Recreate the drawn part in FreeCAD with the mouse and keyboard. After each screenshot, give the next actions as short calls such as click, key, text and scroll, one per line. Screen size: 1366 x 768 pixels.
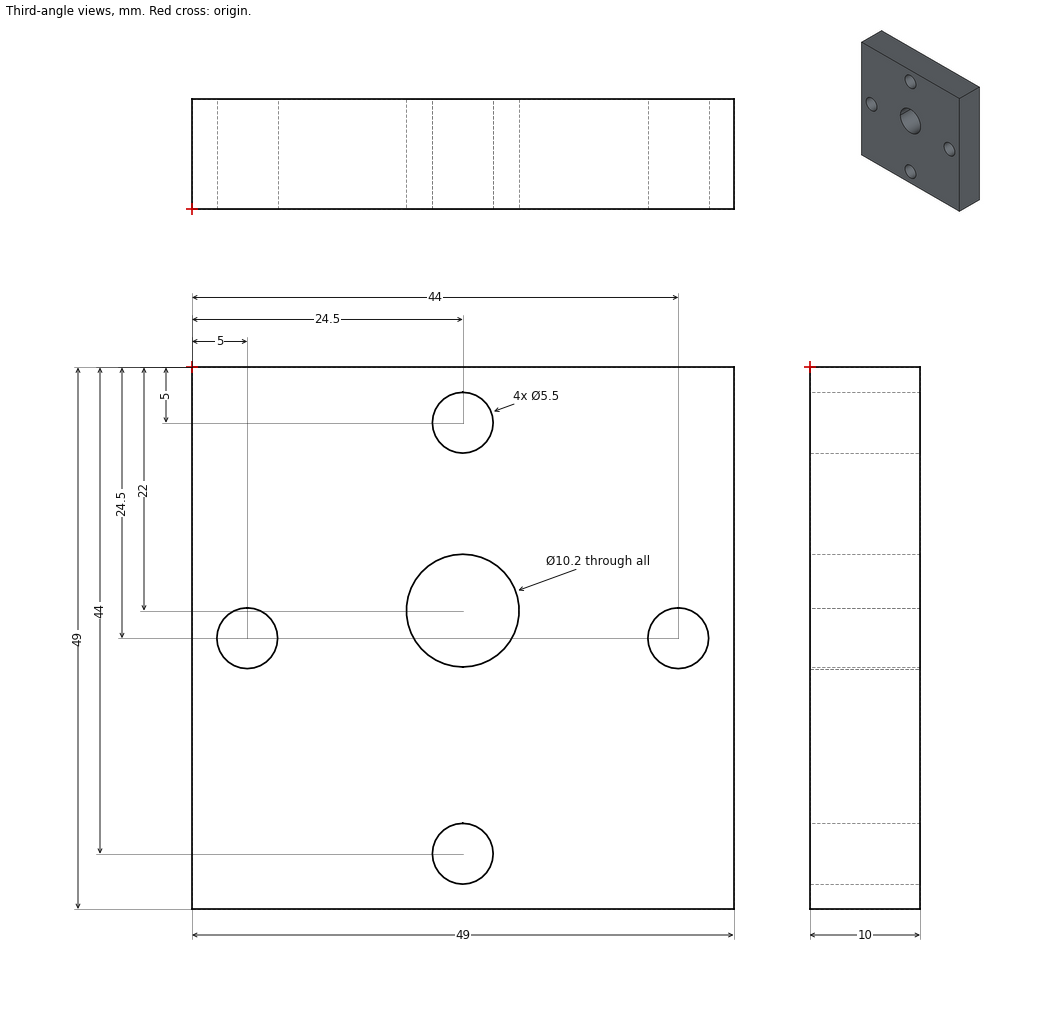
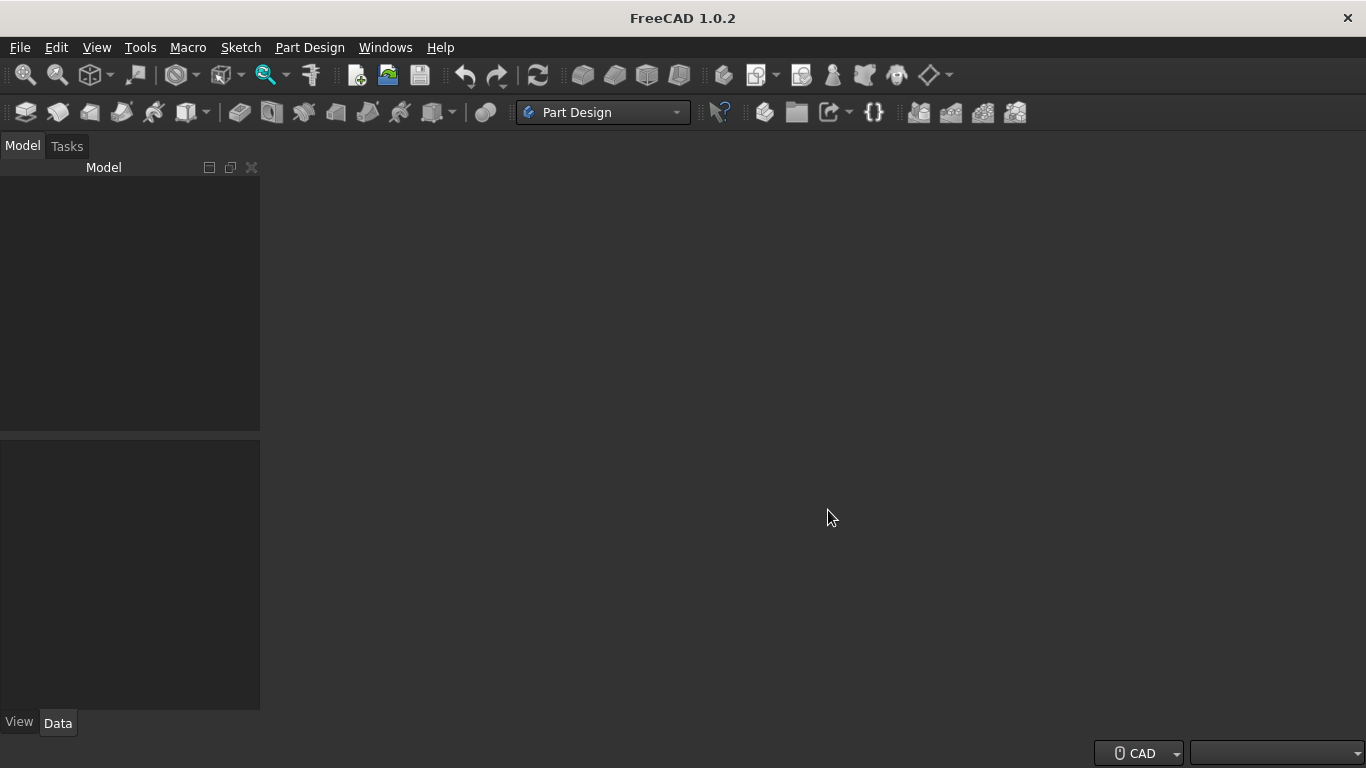
click(356, 76)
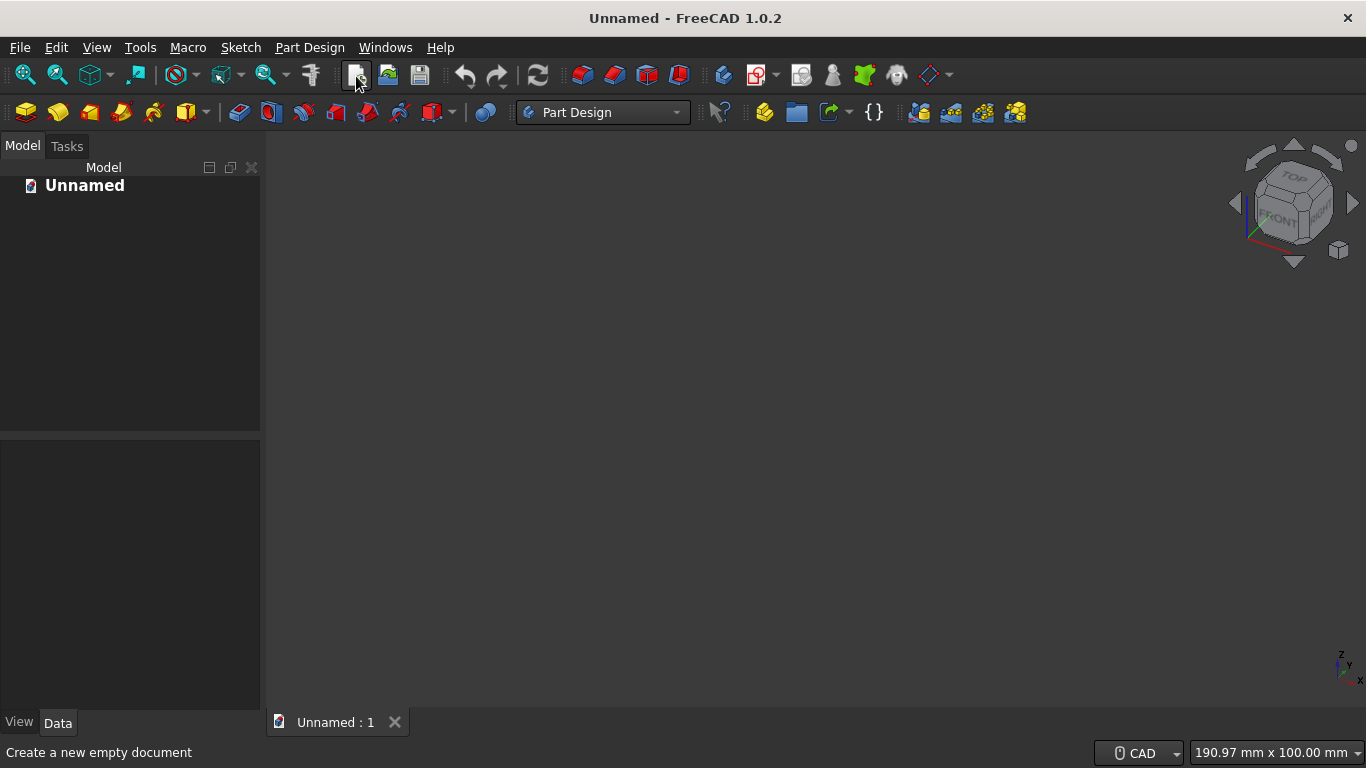
click(756, 76)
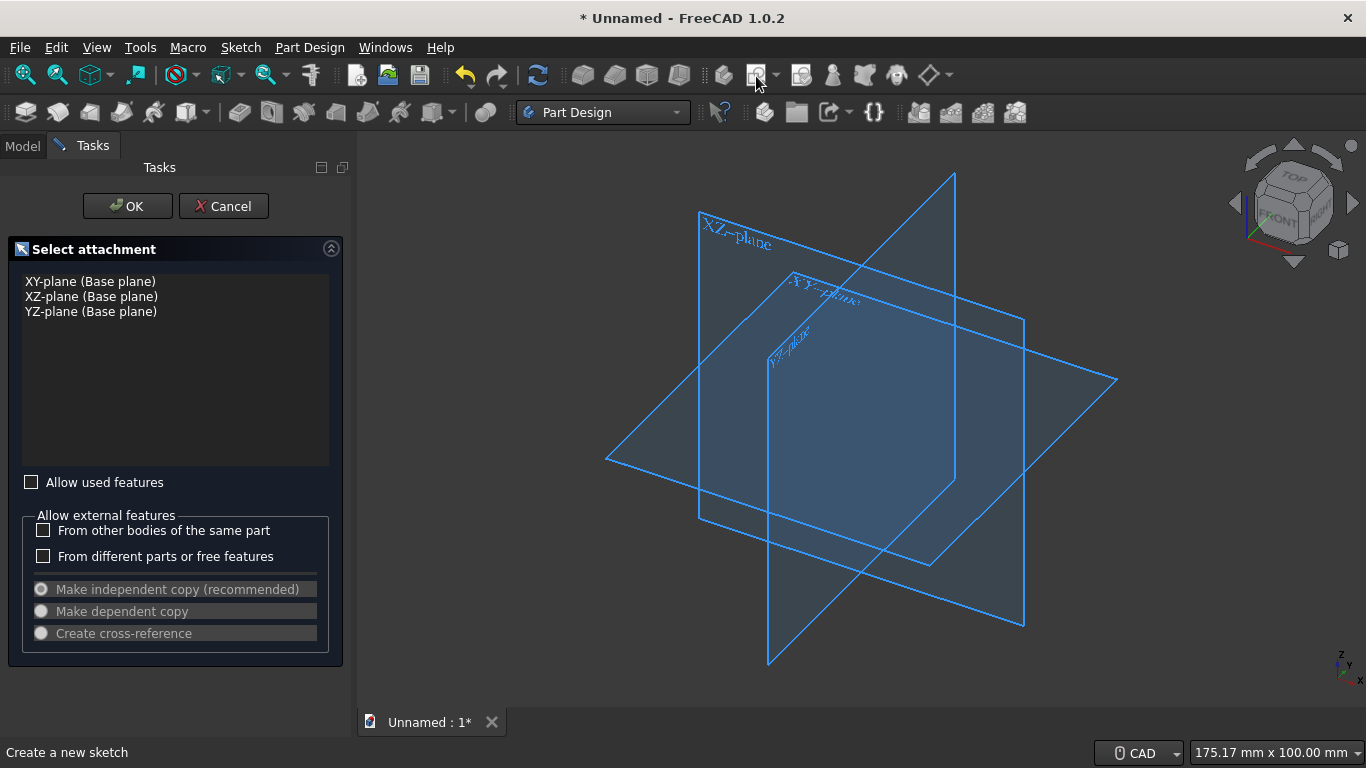
click(82, 296)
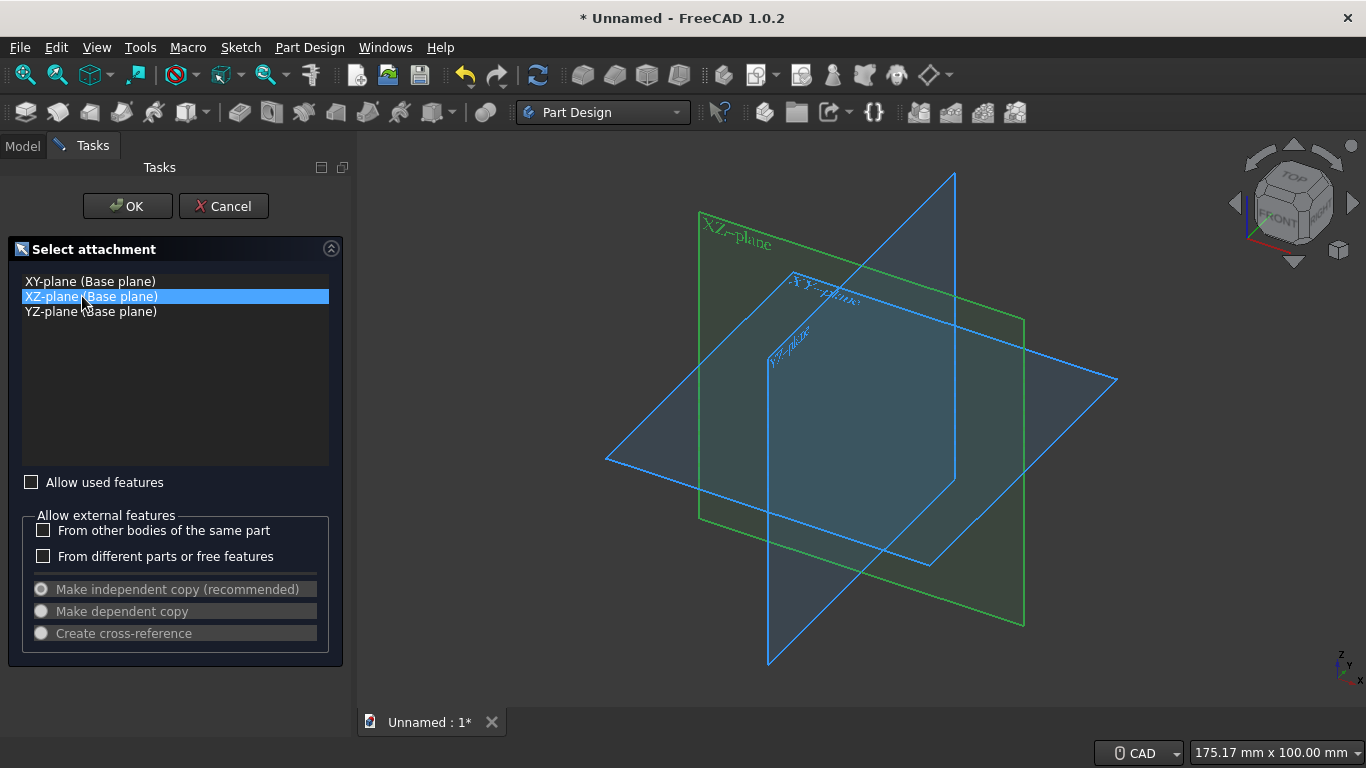
click(128, 206)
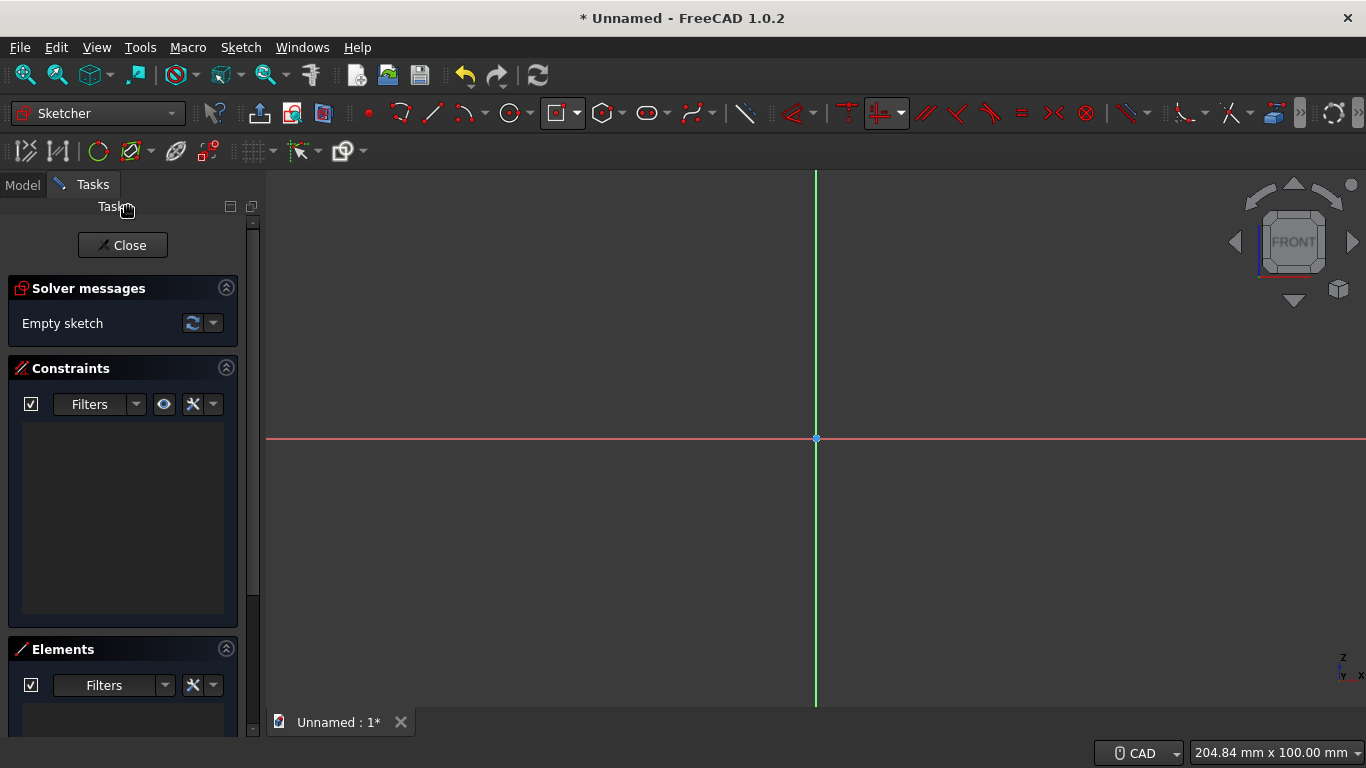
scroll(294, 198, down, 1)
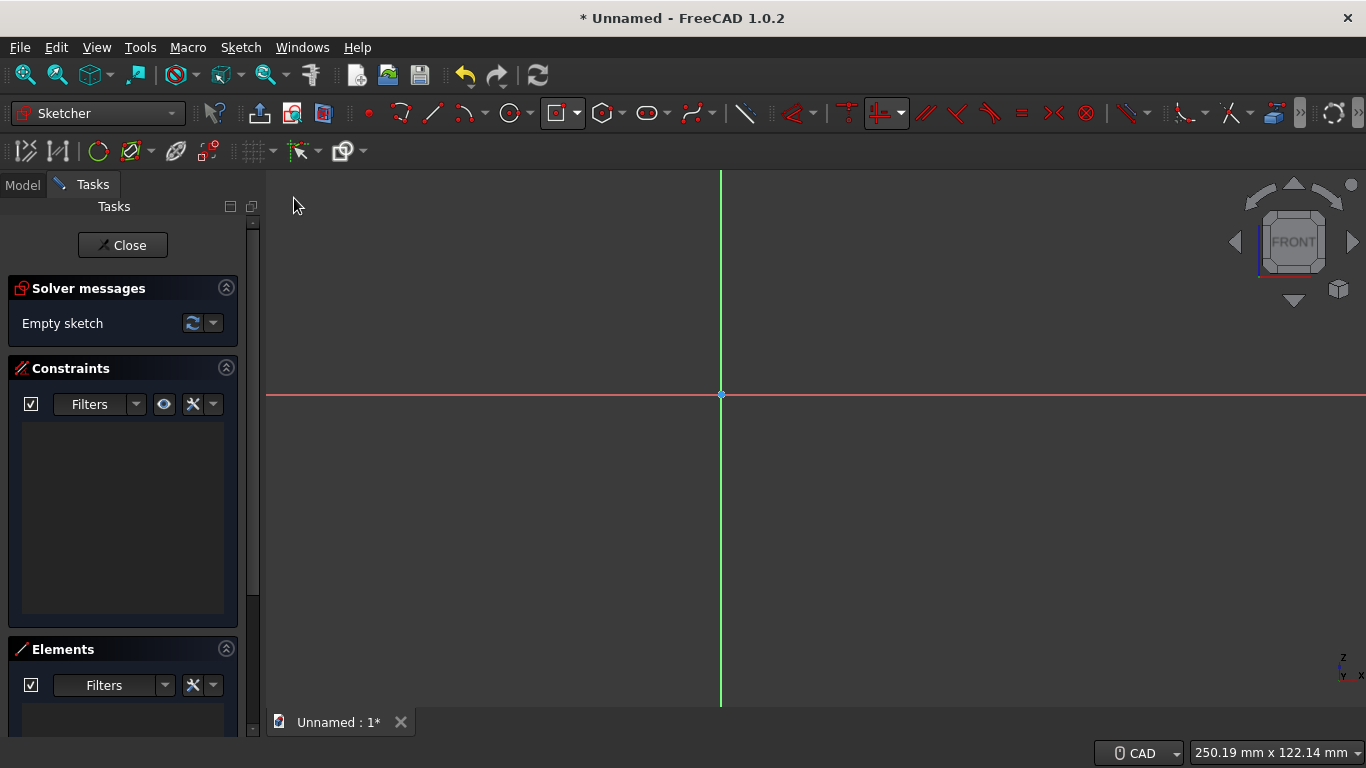
scroll(995, 633, up, 2)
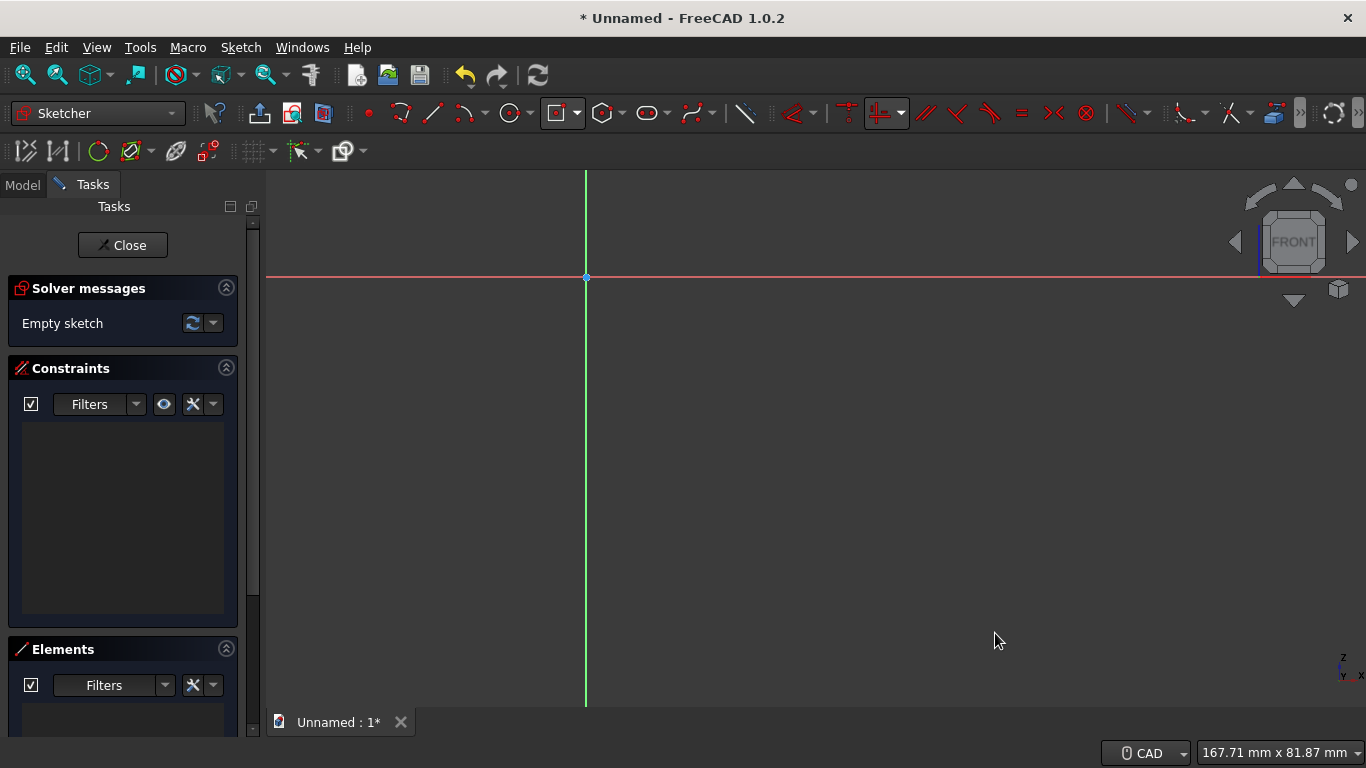
key(g)
key(r)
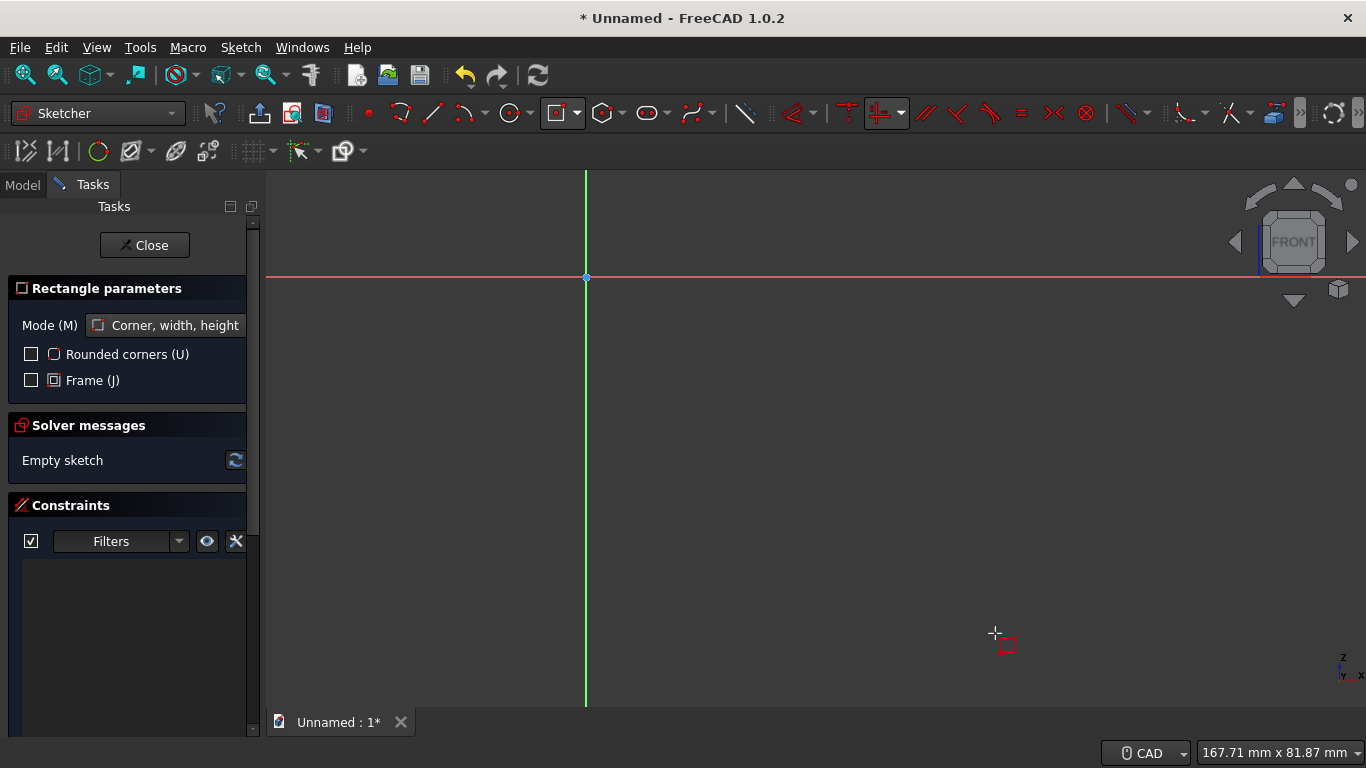
click(586, 277)
click(908, 599)
key(Escape)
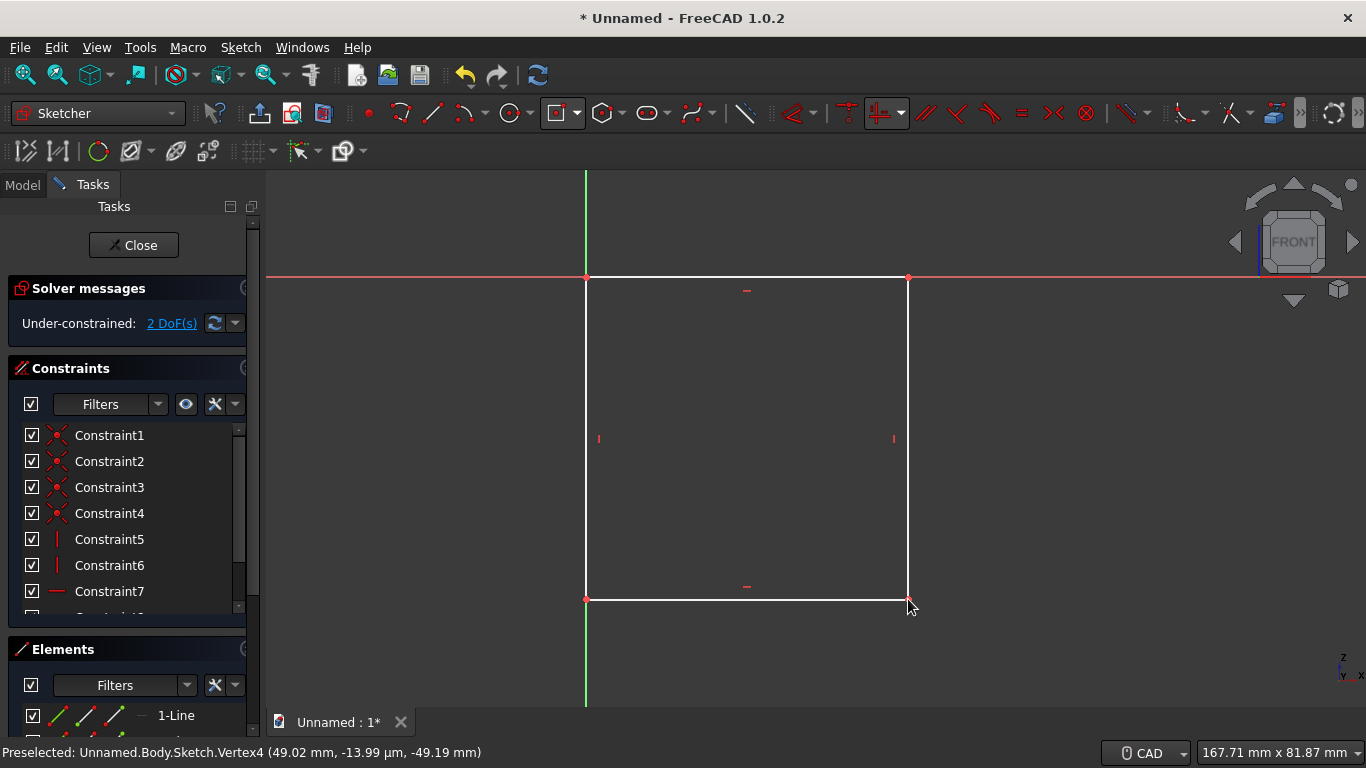
click(792, 114)